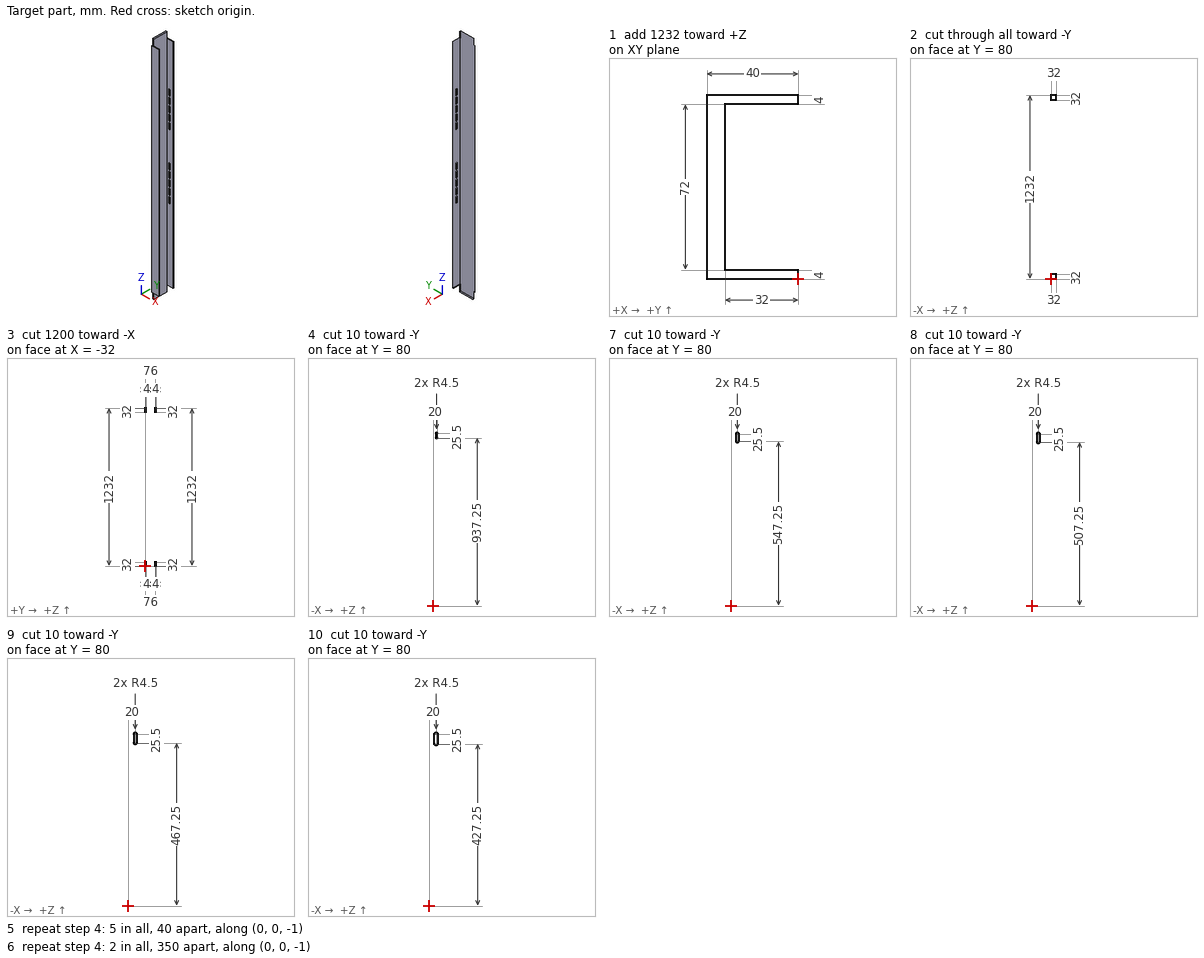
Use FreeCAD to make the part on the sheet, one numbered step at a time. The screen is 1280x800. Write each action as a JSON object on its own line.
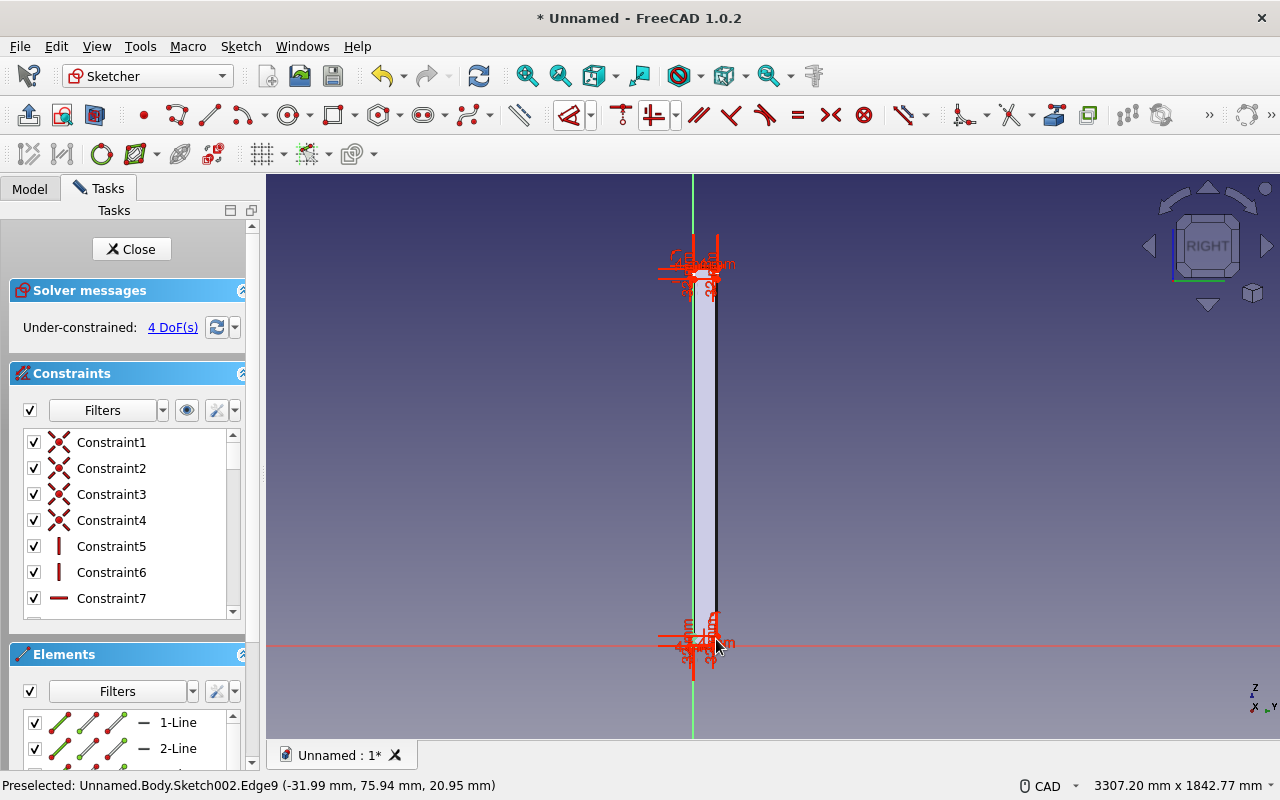
{"action": "scroll", "coordinate": [717, 269], "scroll_direction": "up", "scroll_amount": 12}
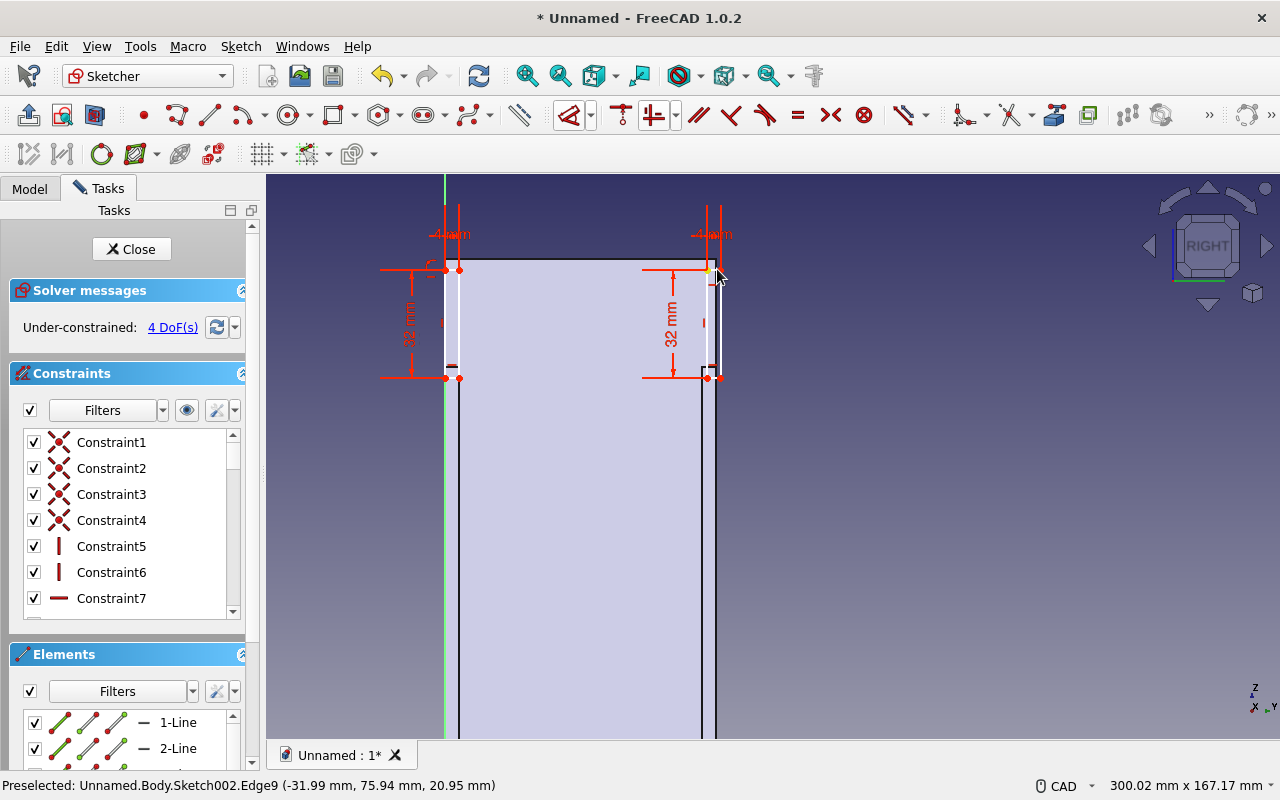
{"action": "left_click", "coordinate": [707, 270]}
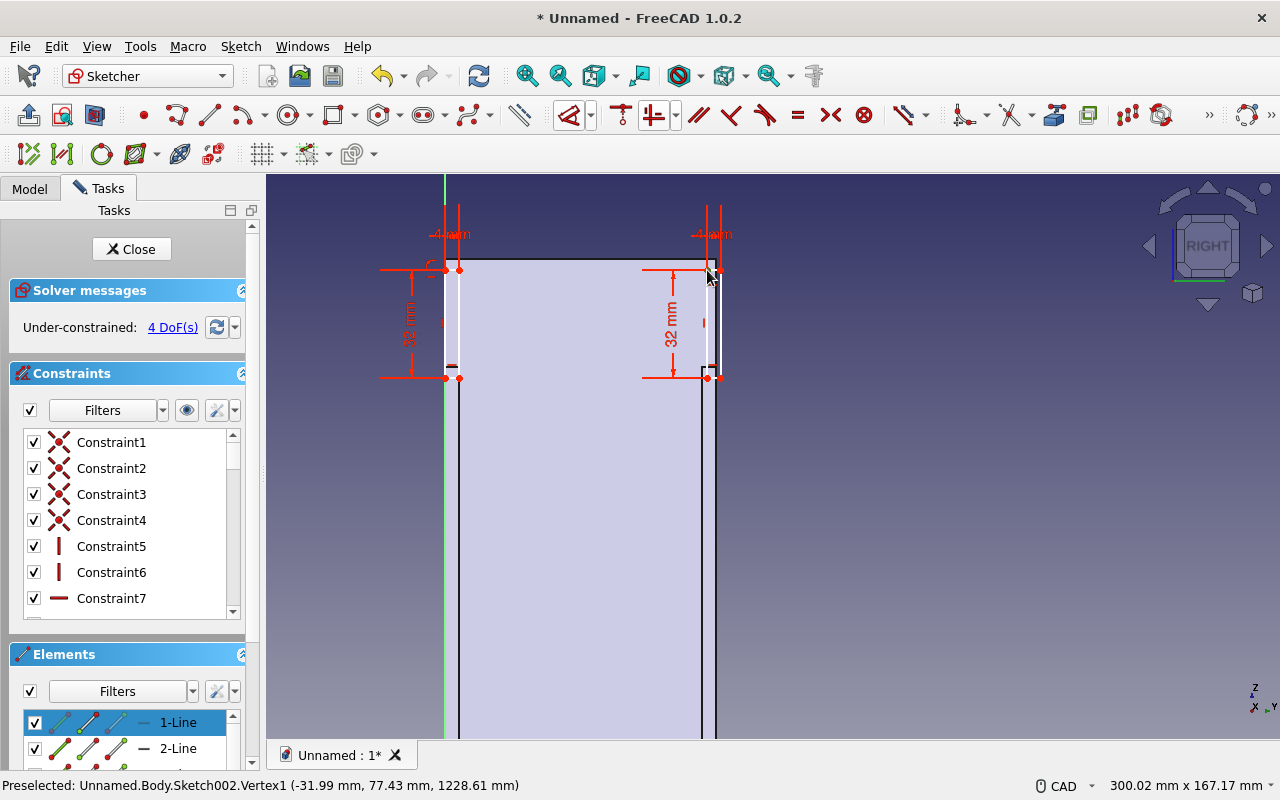
{"action": "key", "text": "l"}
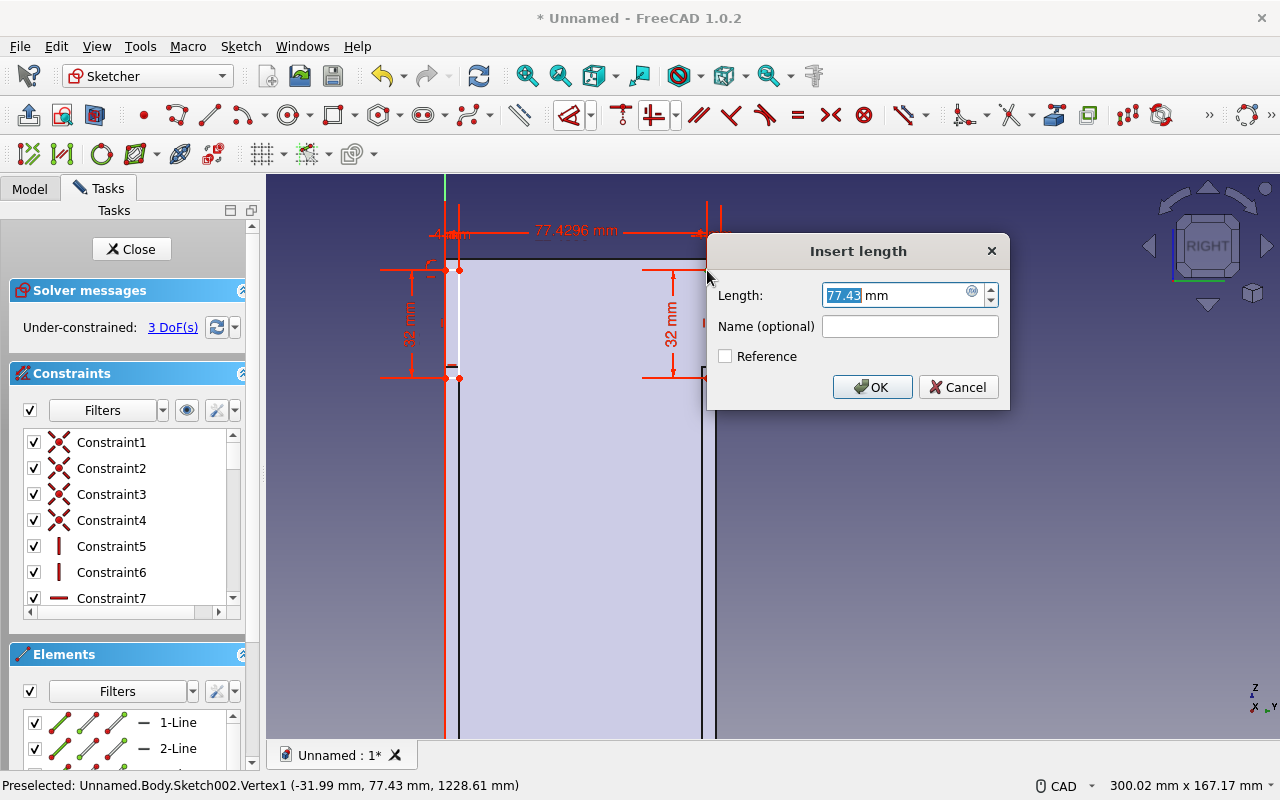
{"action": "type", "text": "76"}
{"action": "key", "text": "Return"}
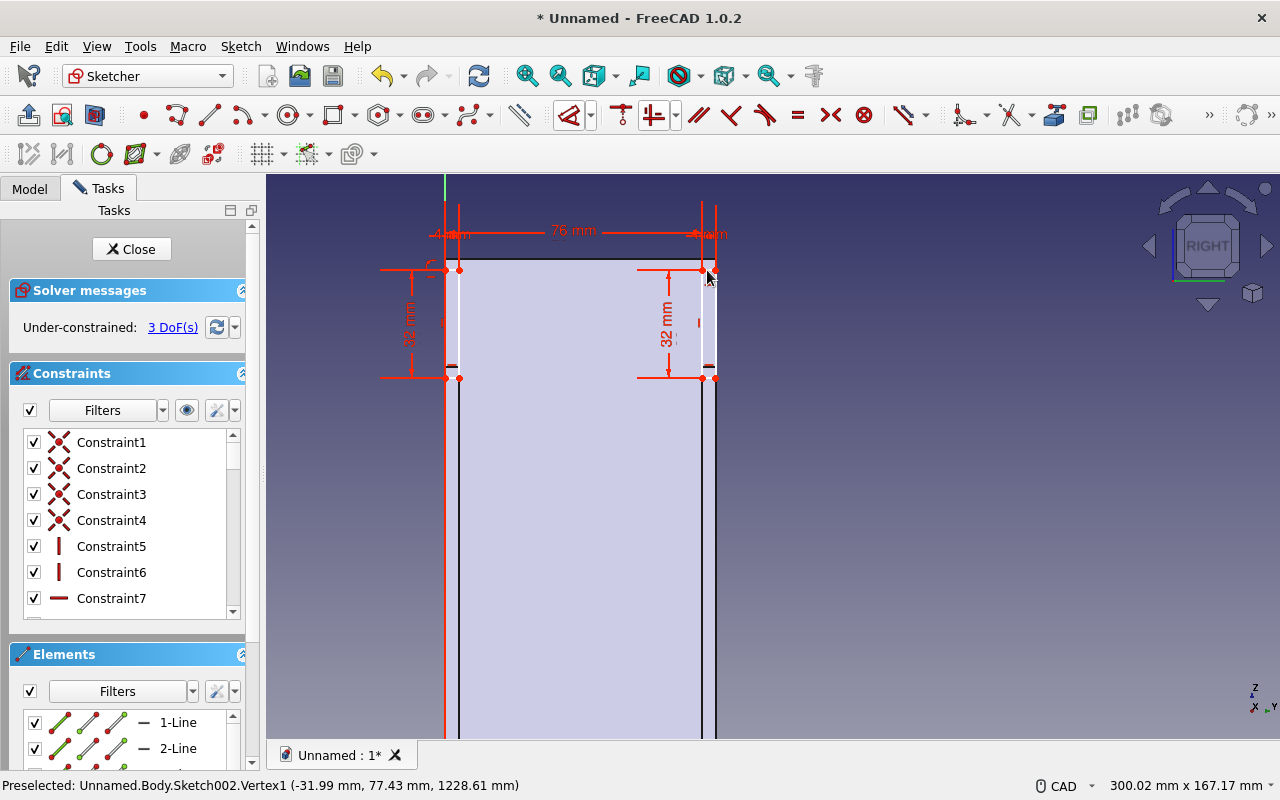
{"action": "scroll", "coordinate": [717, 269], "scroll_direction": "down", "scroll_amount": 12}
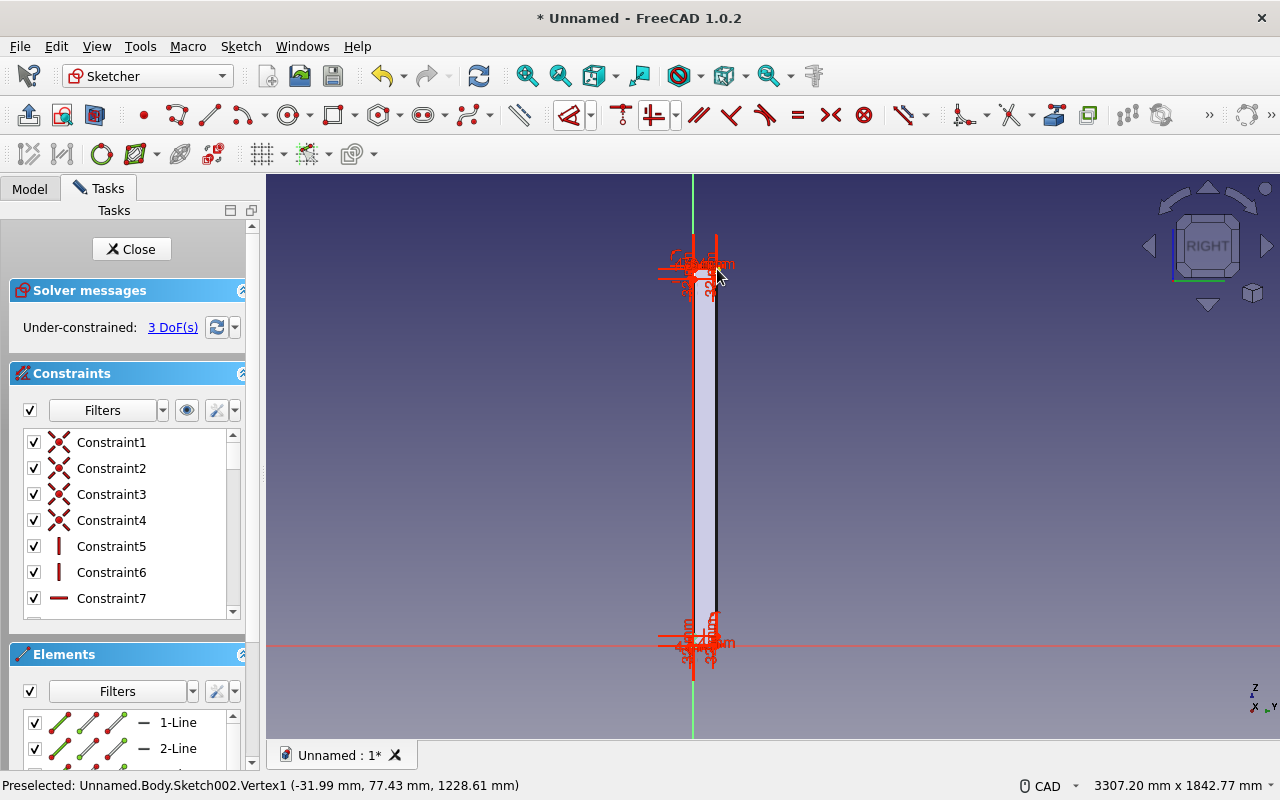
{"action": "scroll", "coordinate": [716, 636], "scroll_direction": "up", "scroll_amount": 12}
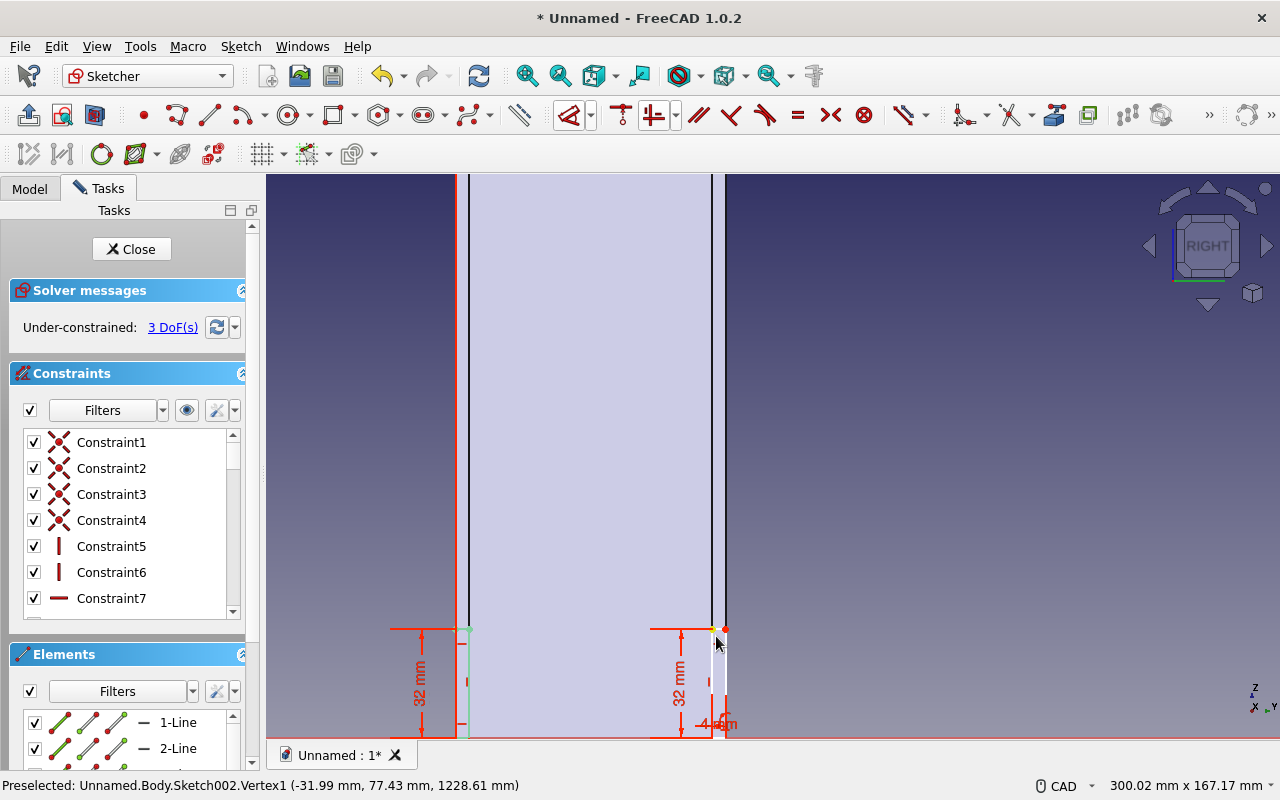
{"action": "left_click", "coordinate": [712, 629]}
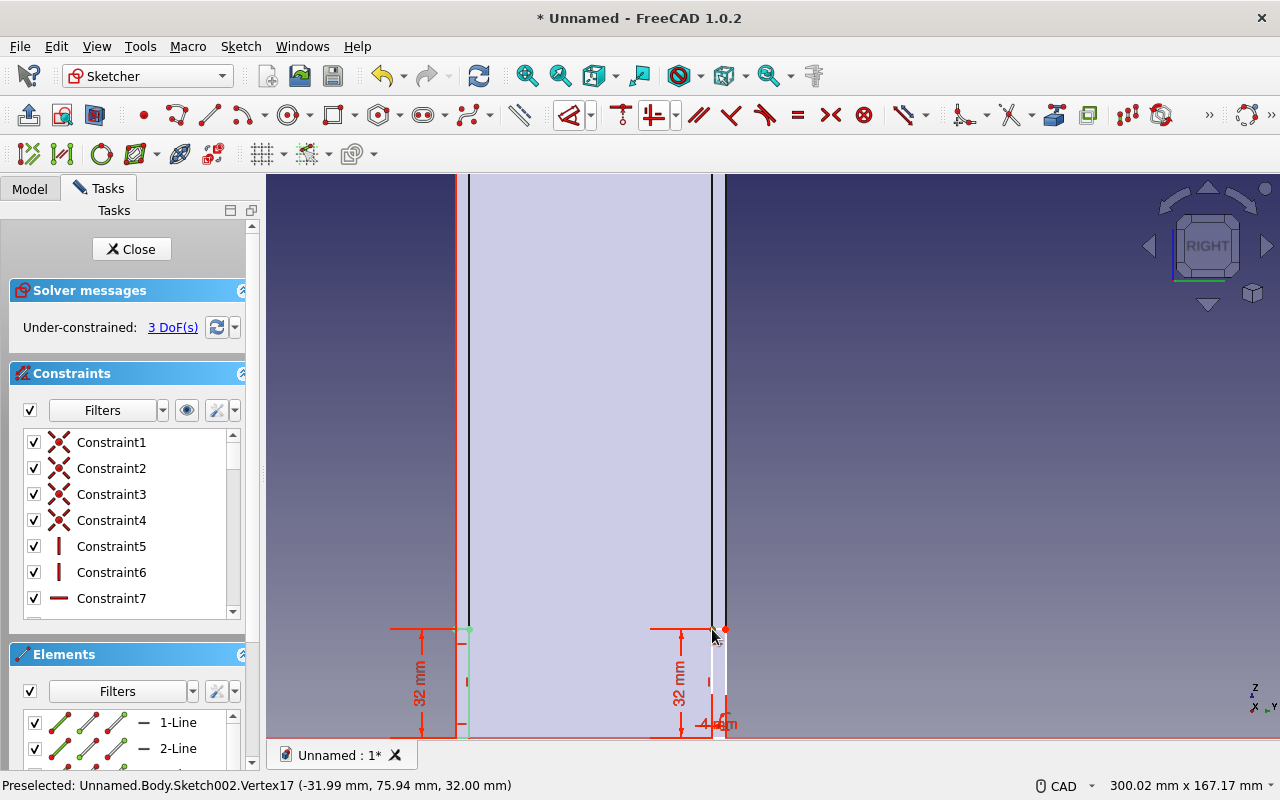
{"action": "left_click", "coordinate": [590, 116]}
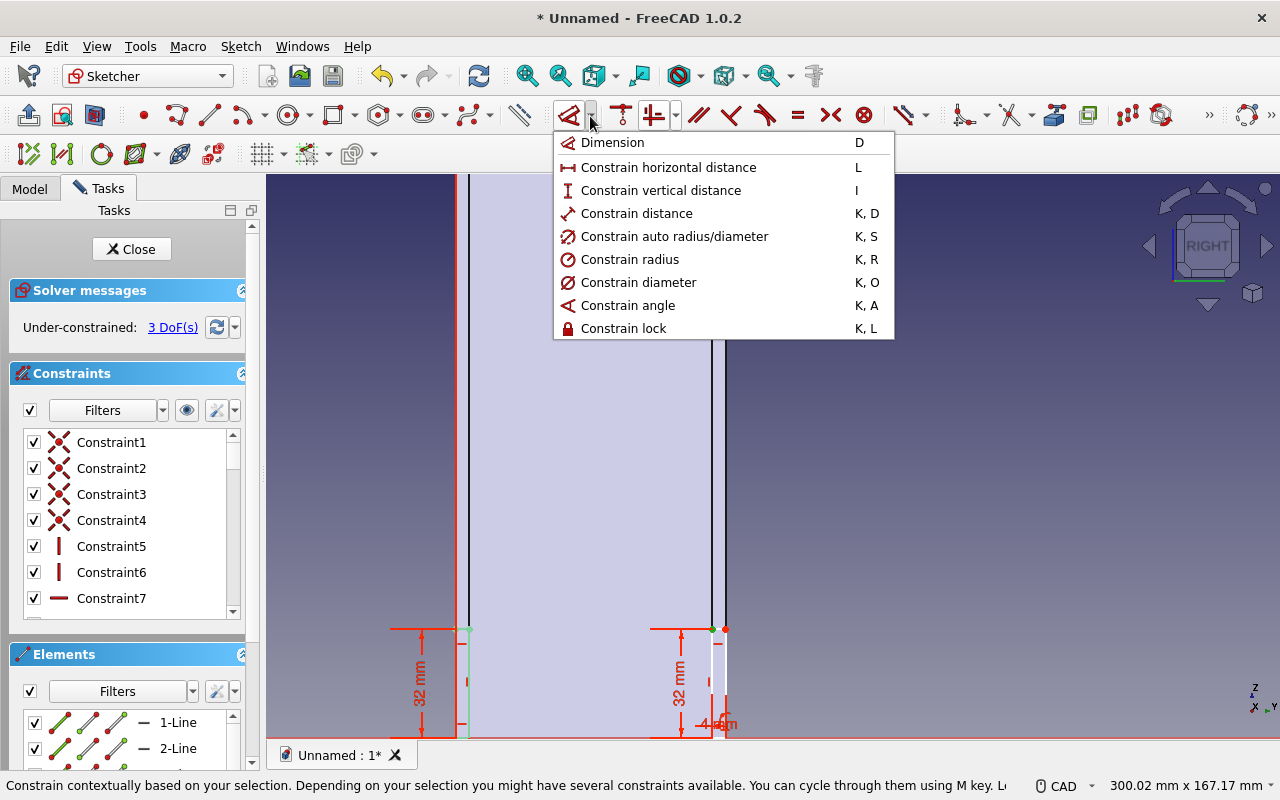
{"action": "left_click", "coordinate": [724, 168]}